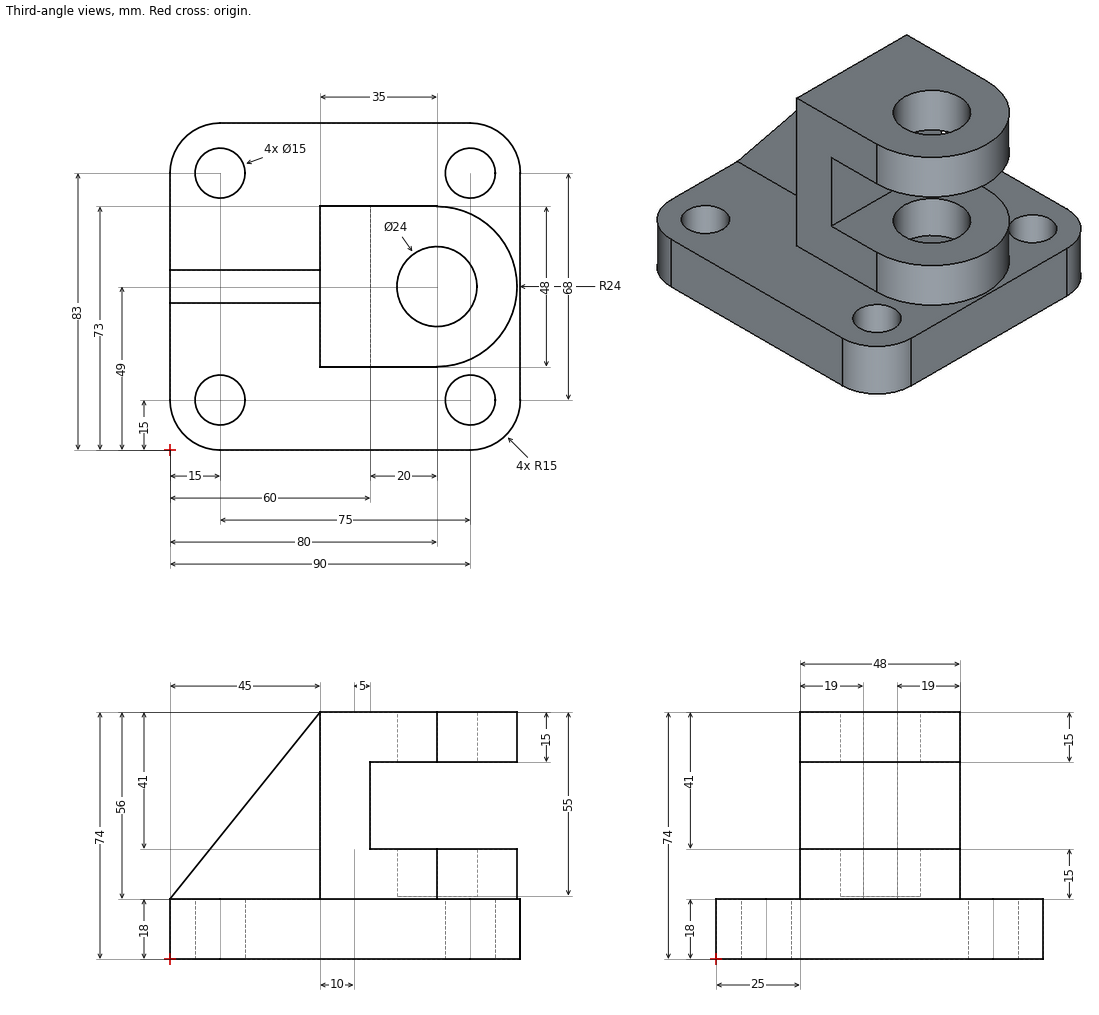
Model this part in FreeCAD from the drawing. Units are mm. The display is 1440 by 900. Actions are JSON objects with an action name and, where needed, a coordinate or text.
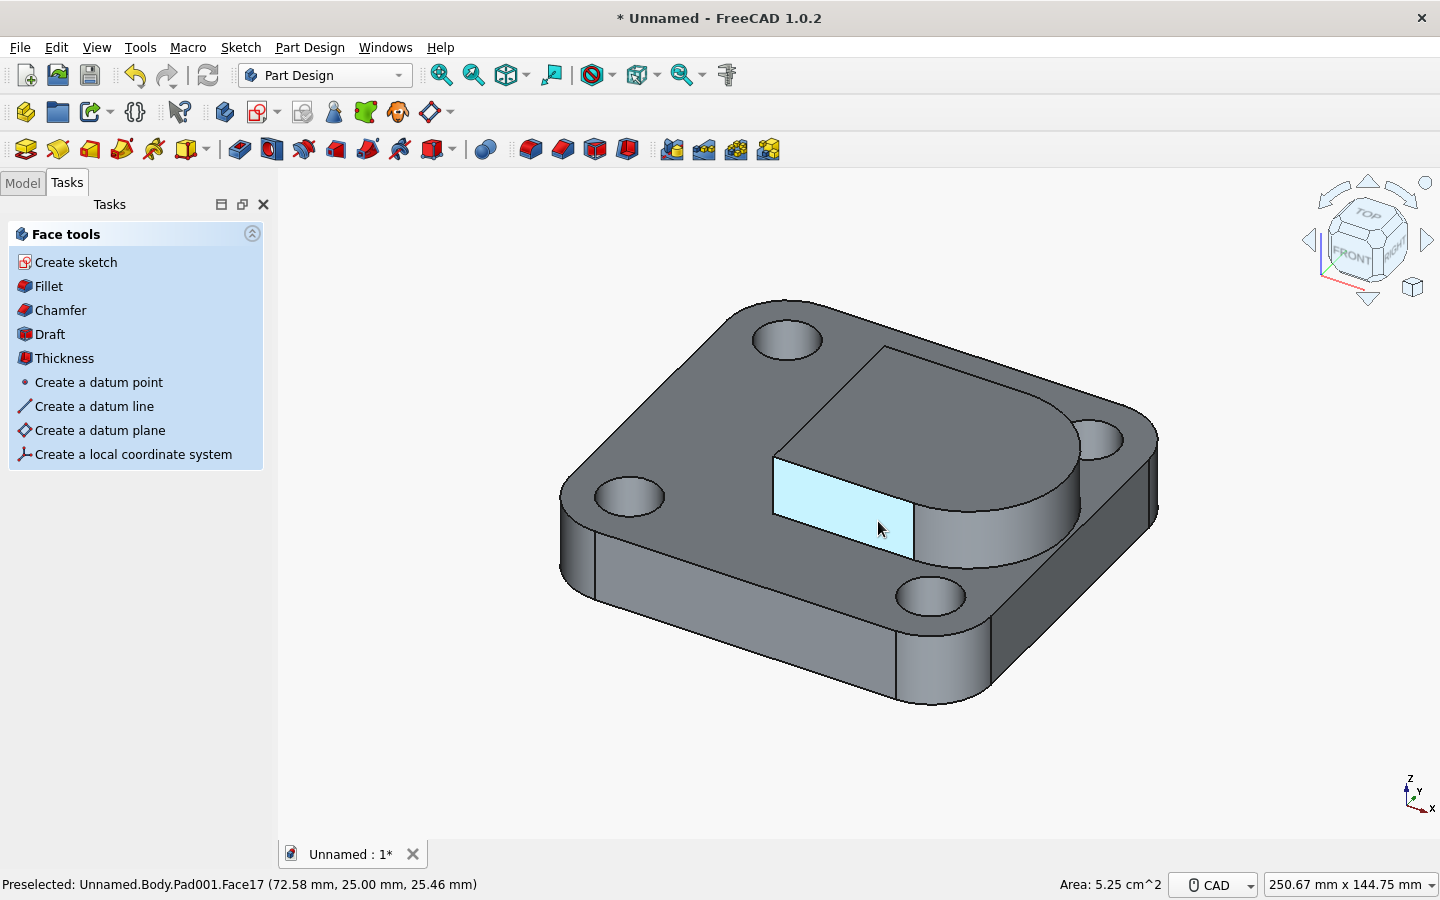
{"action": "left_click", "coordinate": [258, 112]}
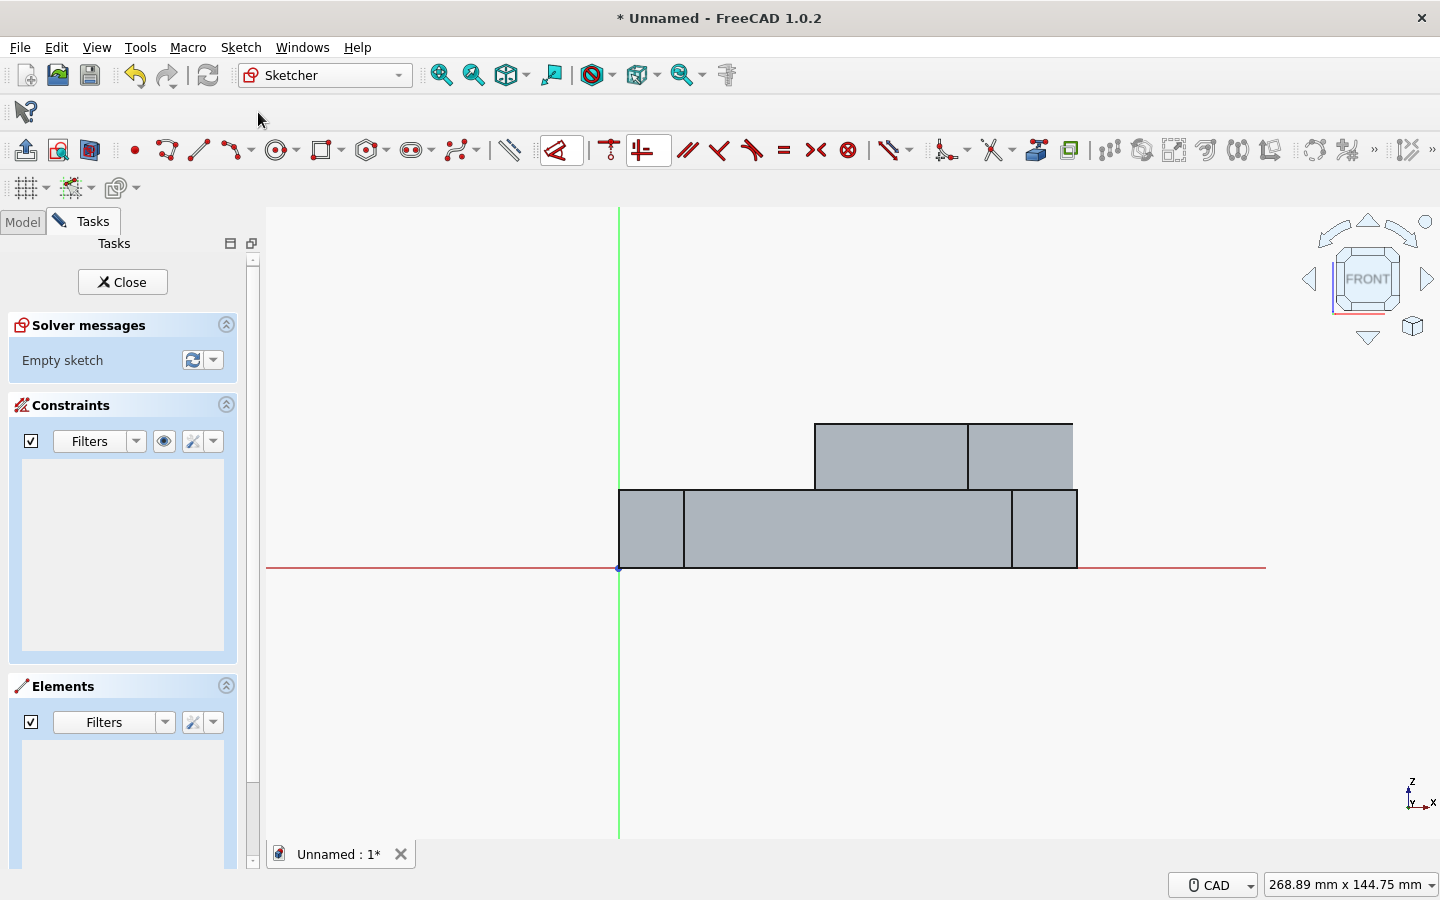
{"action": "left_click", "coordinate": [90, 150]}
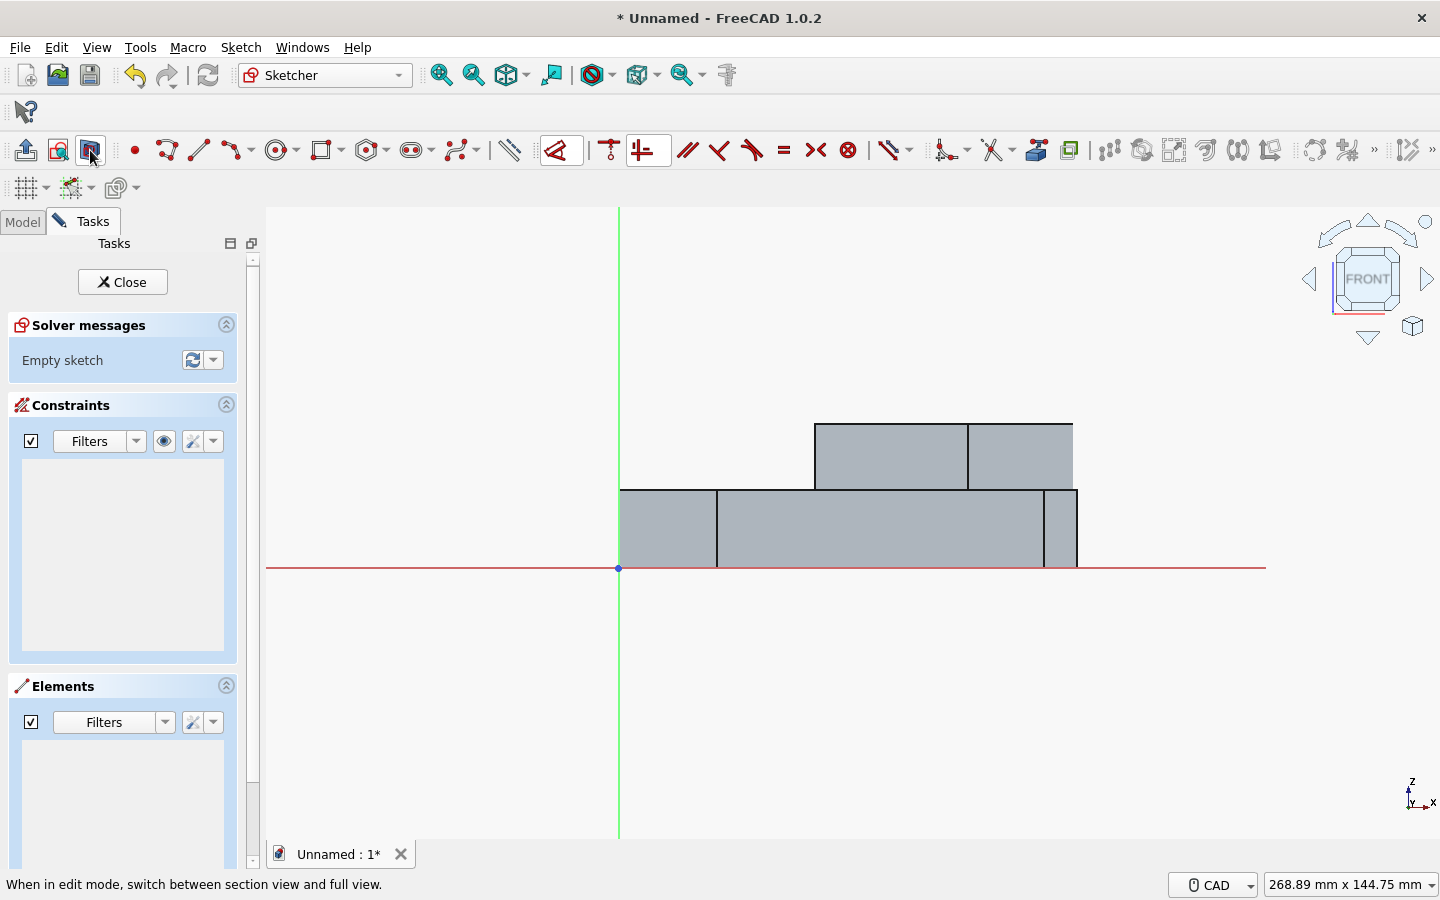
{"action": "scroll", "coordinate": [991, 811], "scroll_direction": "down", "scroll_amount": 1}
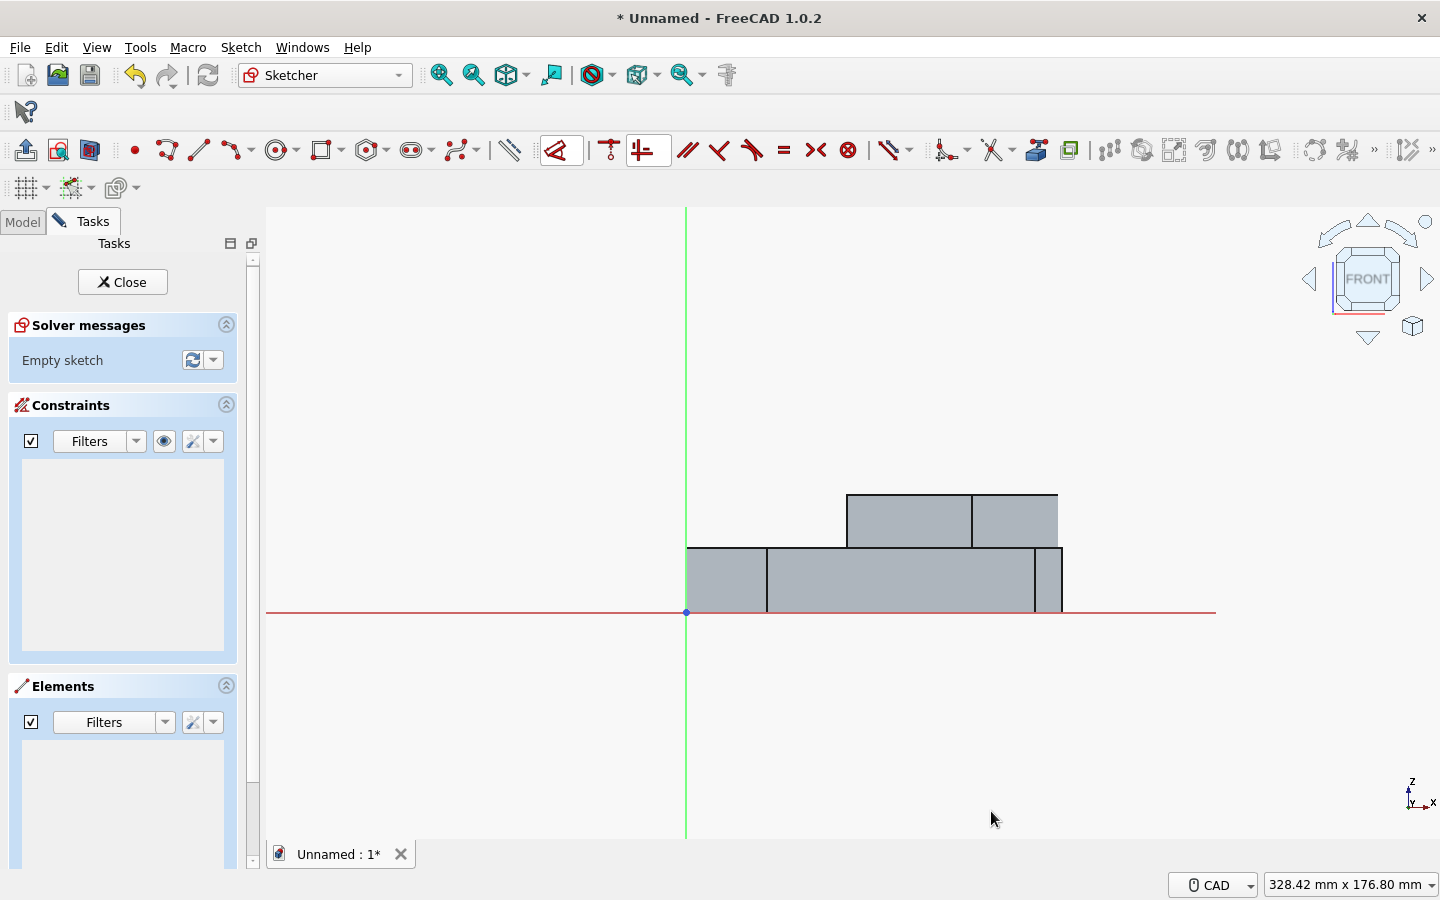
{"action": "scroll", "coordinate": [785, 393], "scroll_direction": "up", "scroll_amount": 2}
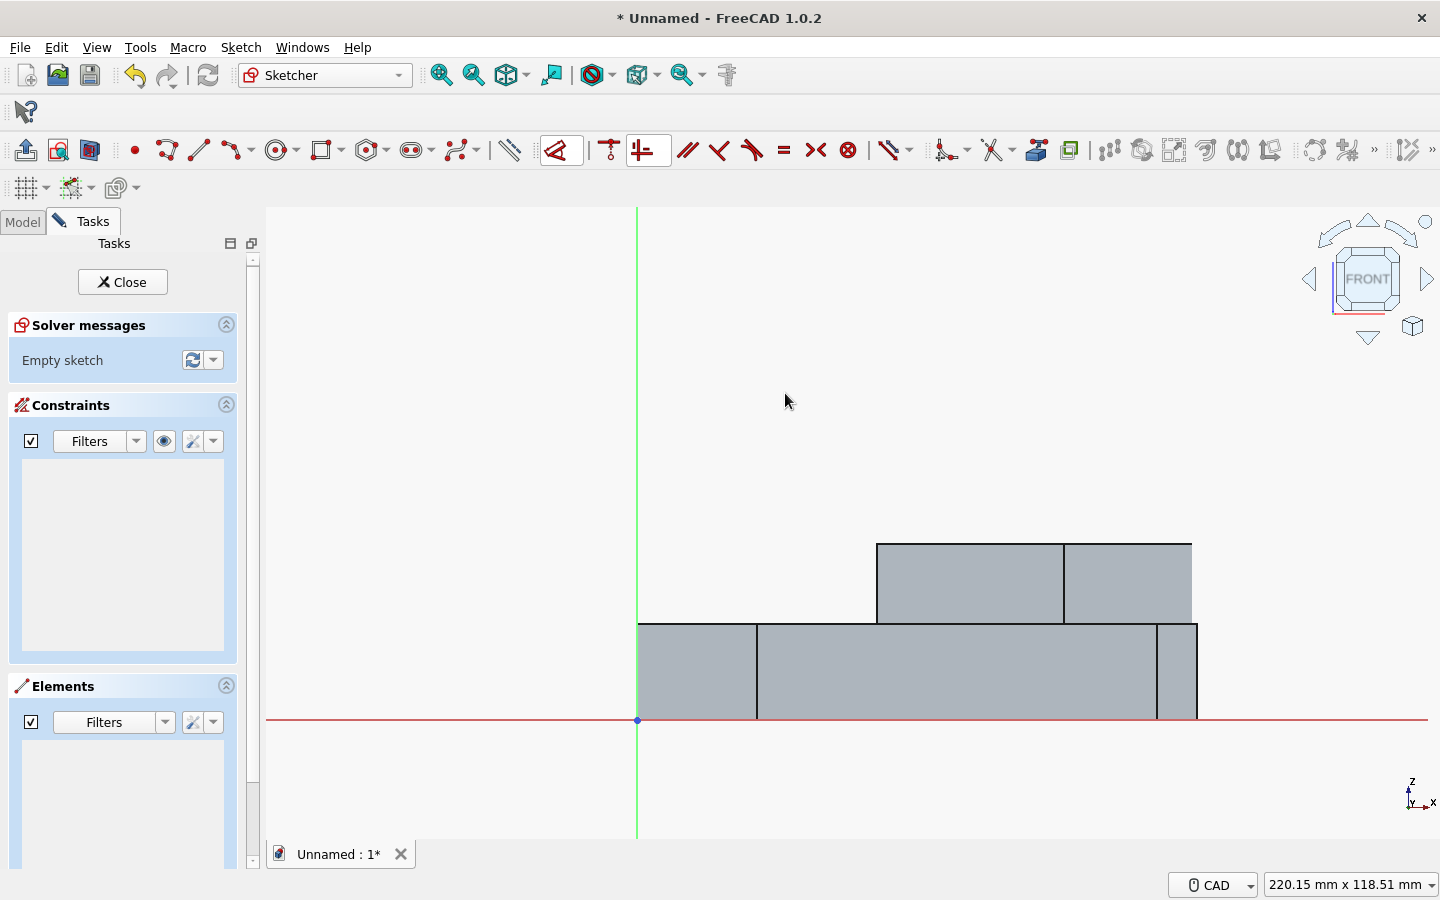
{"action": "left_click", "coordinate": [322, 150]}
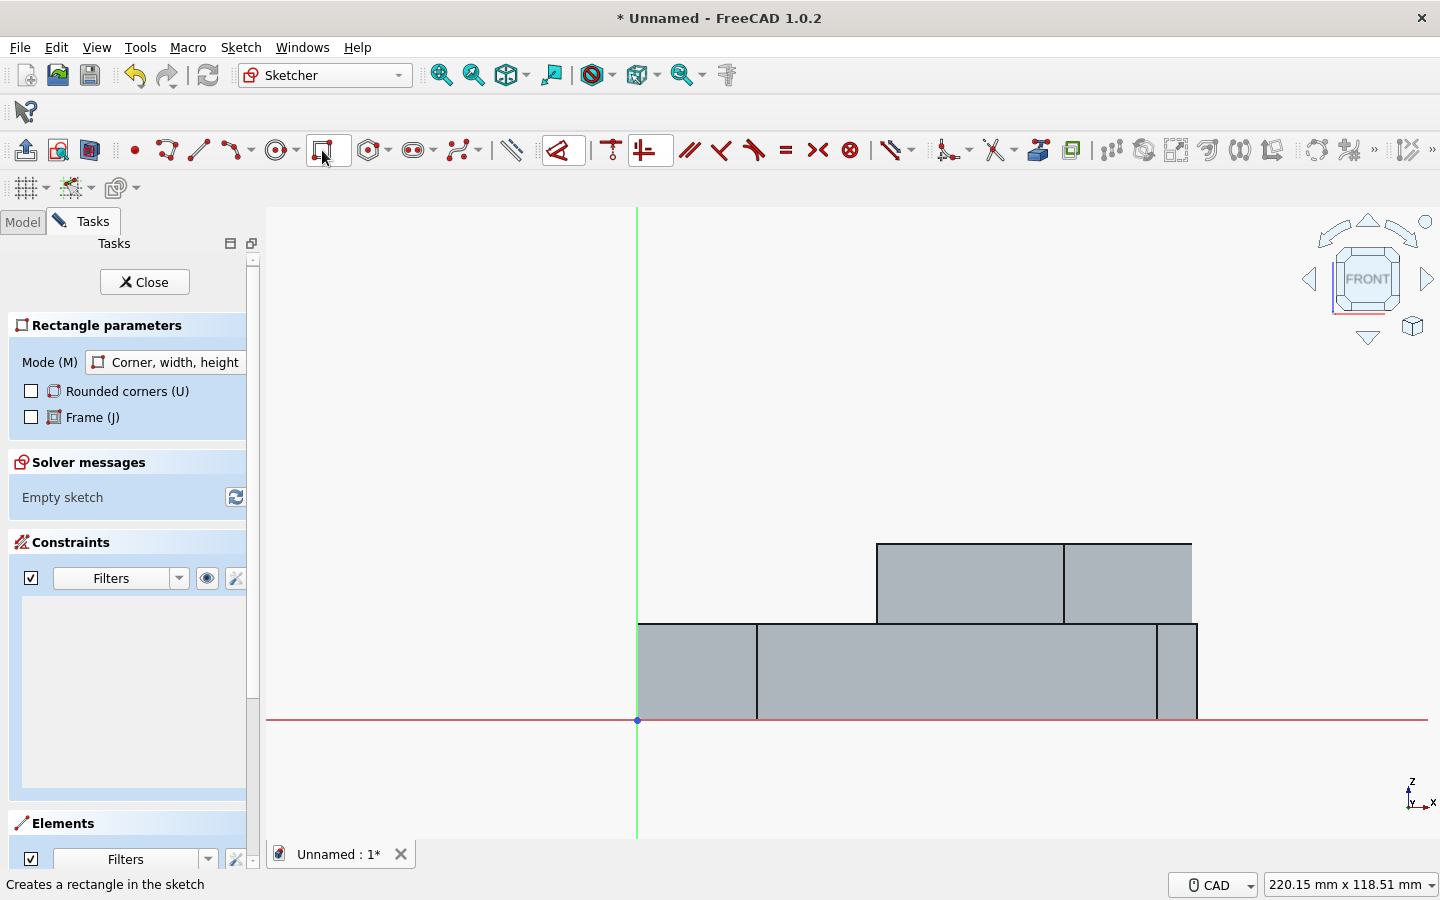
{"action": "left_click", "coordinate": [877, 326]}
{"action": "left_click", "coordinate": [931, 544]}
{"action": "key", "text": "Escape"}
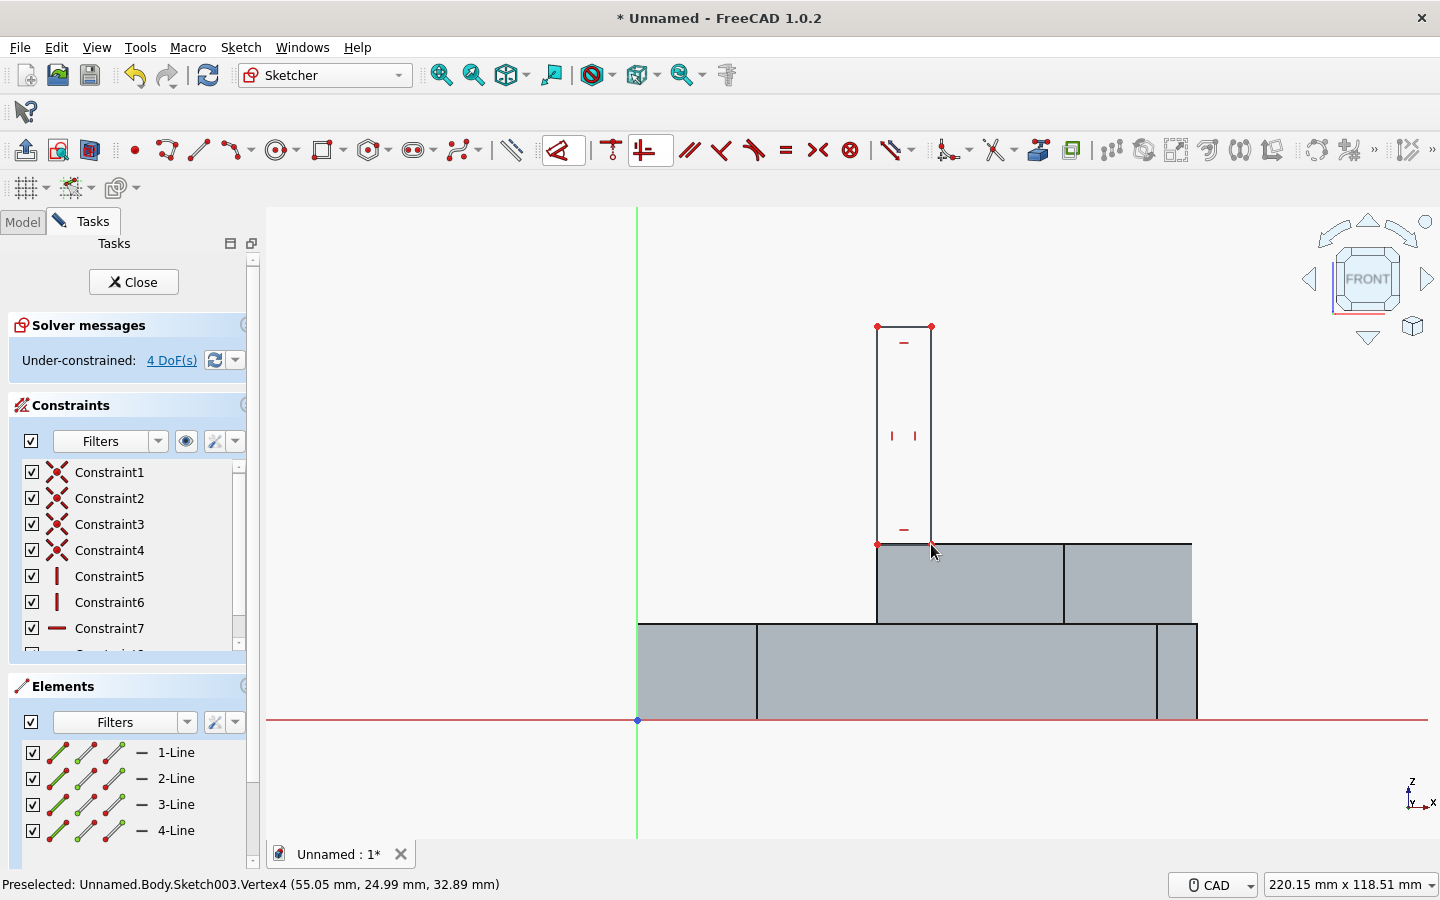
{"action": "left_click", "coordinate": [877, 392]}